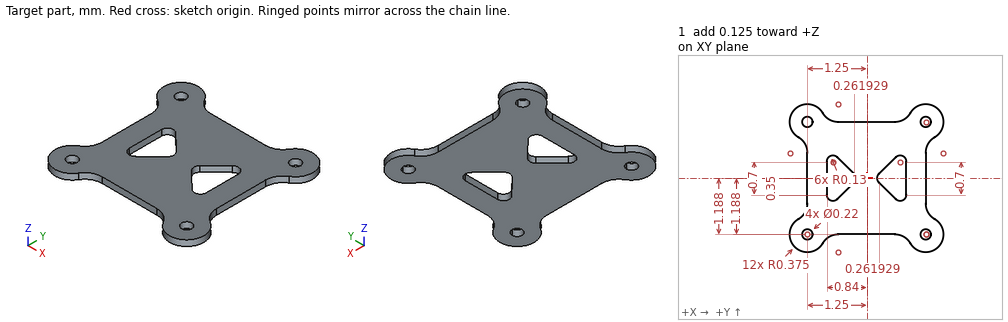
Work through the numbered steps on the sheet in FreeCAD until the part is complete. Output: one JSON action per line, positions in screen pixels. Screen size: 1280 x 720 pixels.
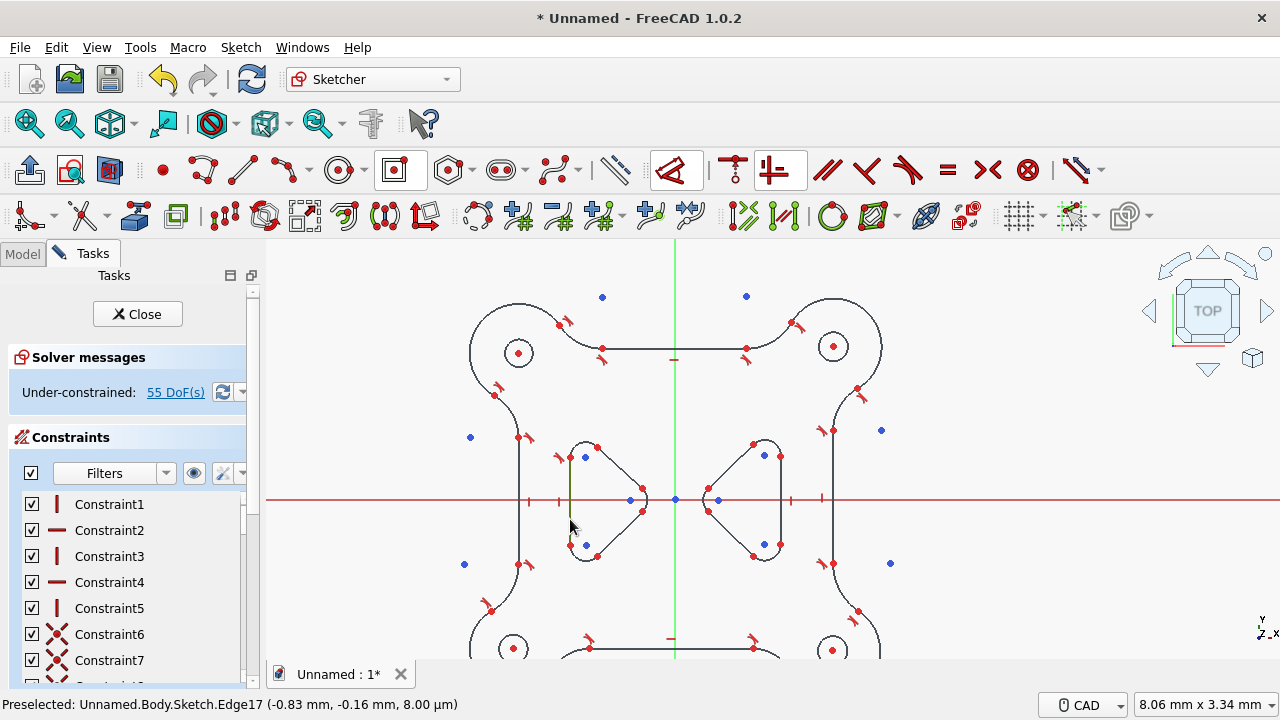
{"action": "scroll", "coordinate": [574, 556], "scroll_direction": "up", "scroll_amount": 2}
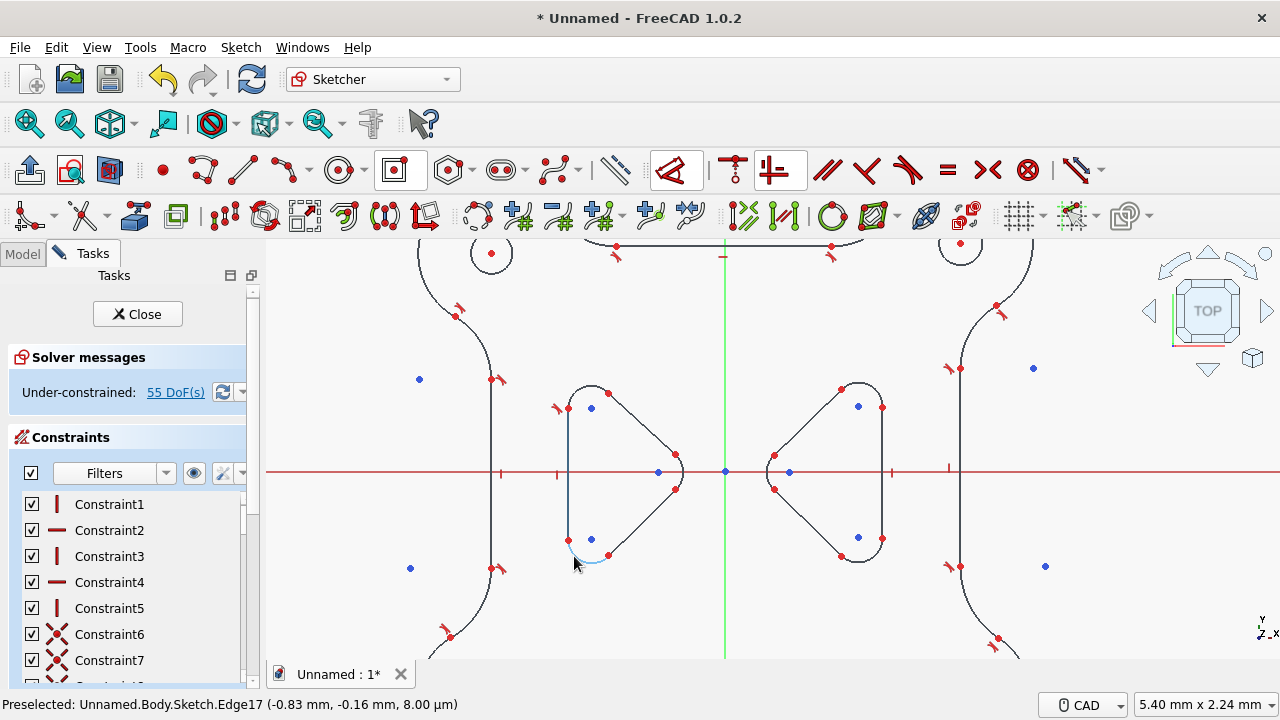
{"action": "left_click", "coordinate": [574, 555]}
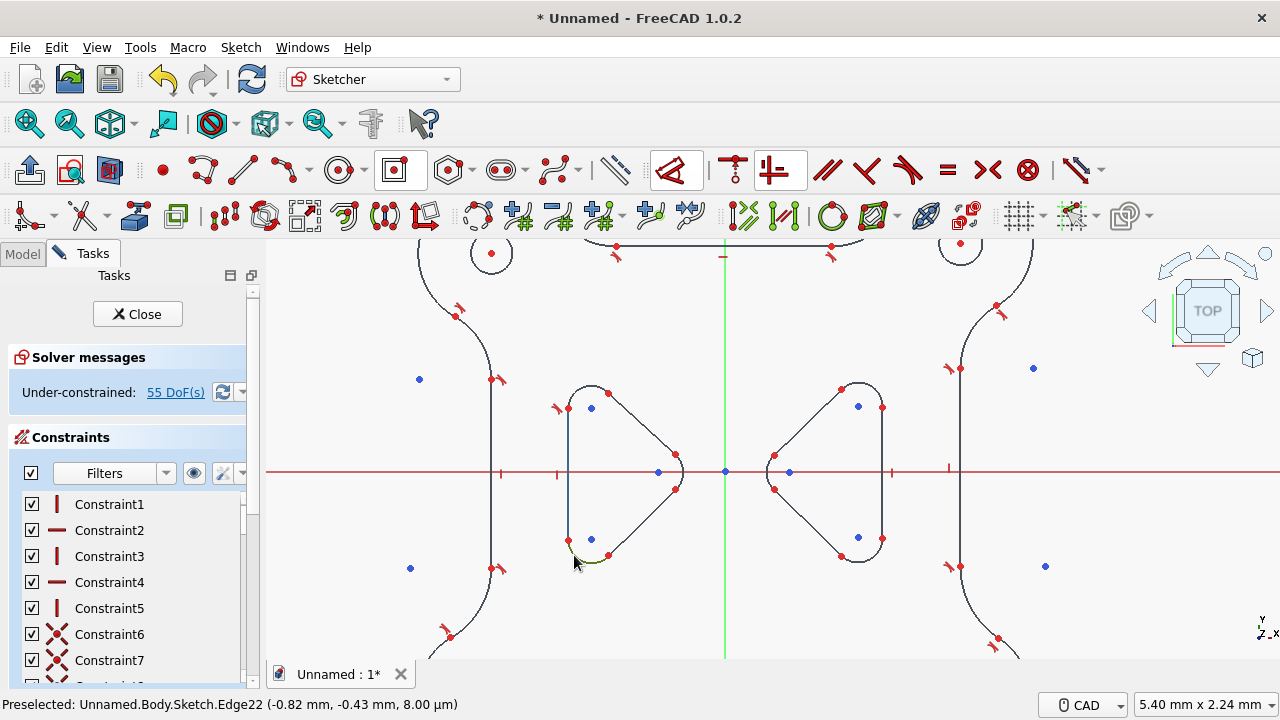
{"action": "left_click", "coordinate": [908, 170]}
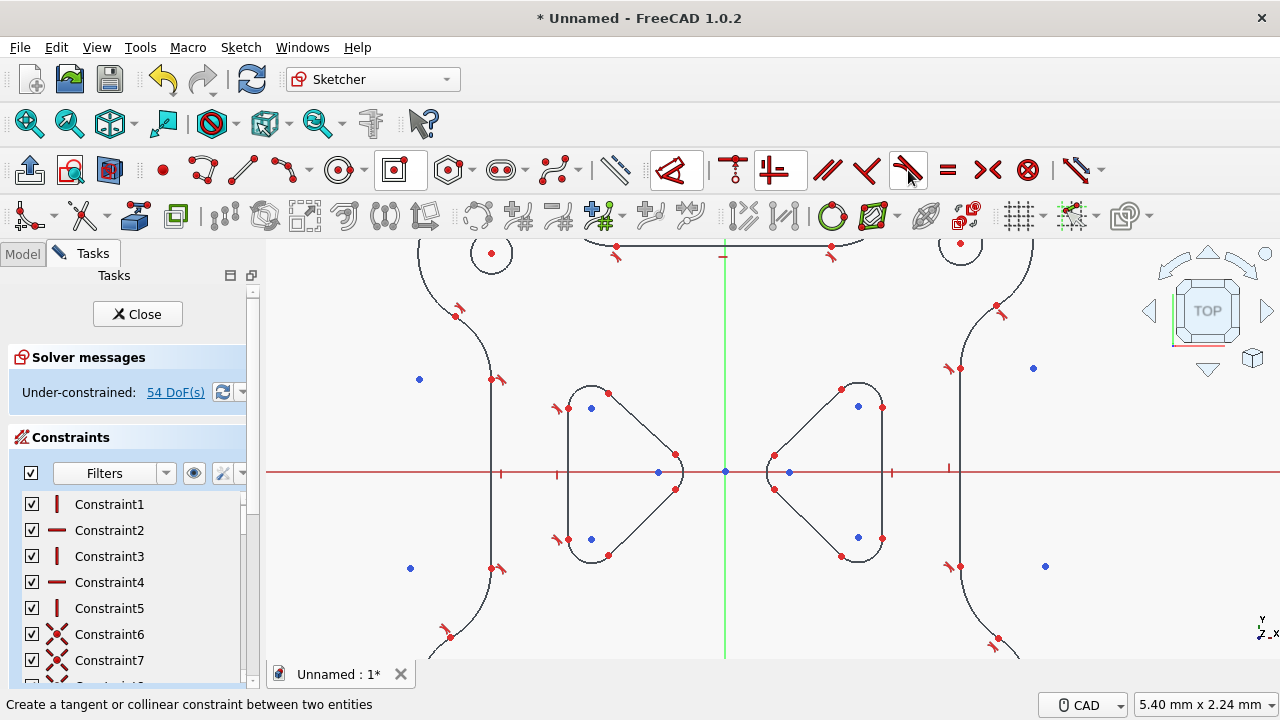
{"action": "left_click", "coordinate": [629, 412]}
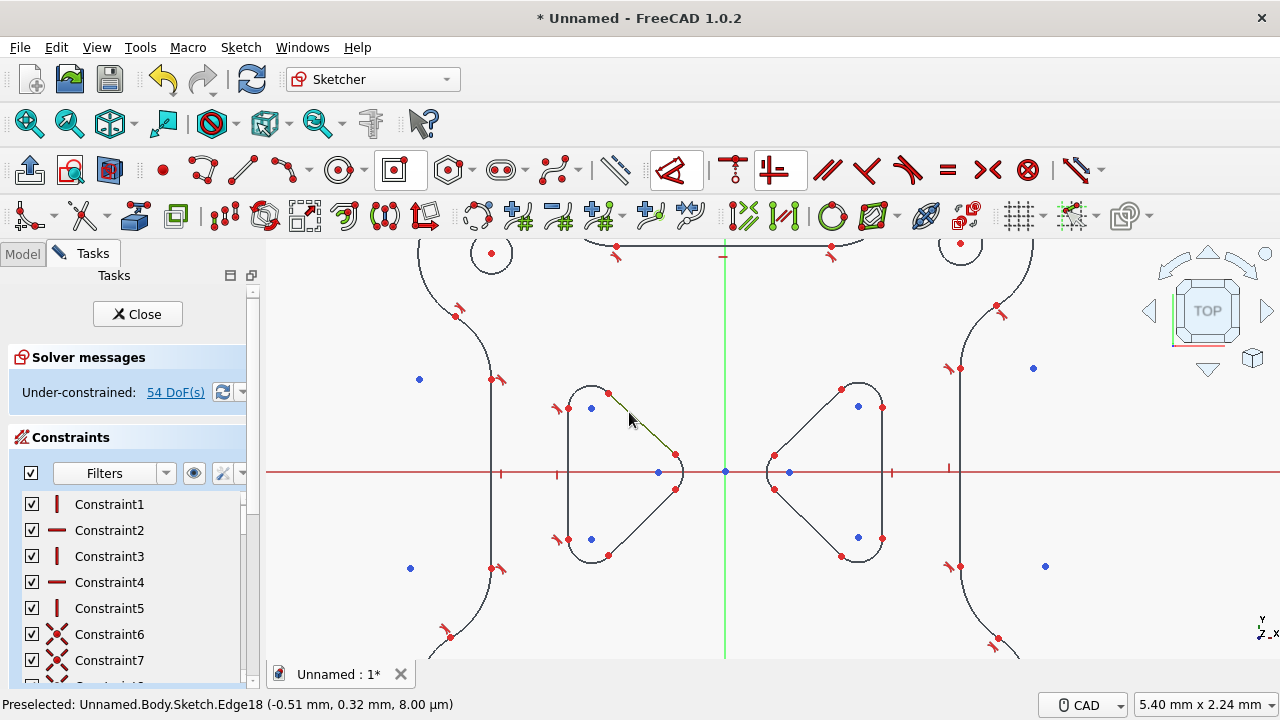
{"action": "left_click", "coordinate": [594, 386]}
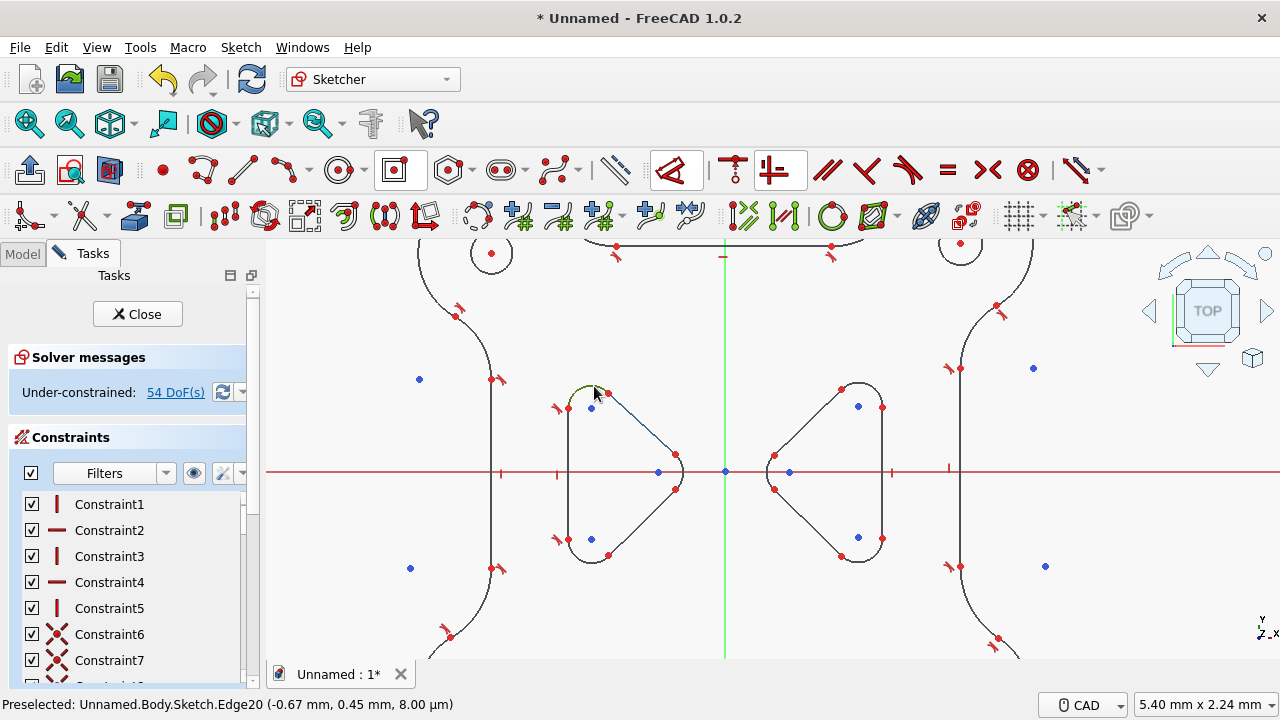
{"action": "left_click", "coordinate": [908, 170]}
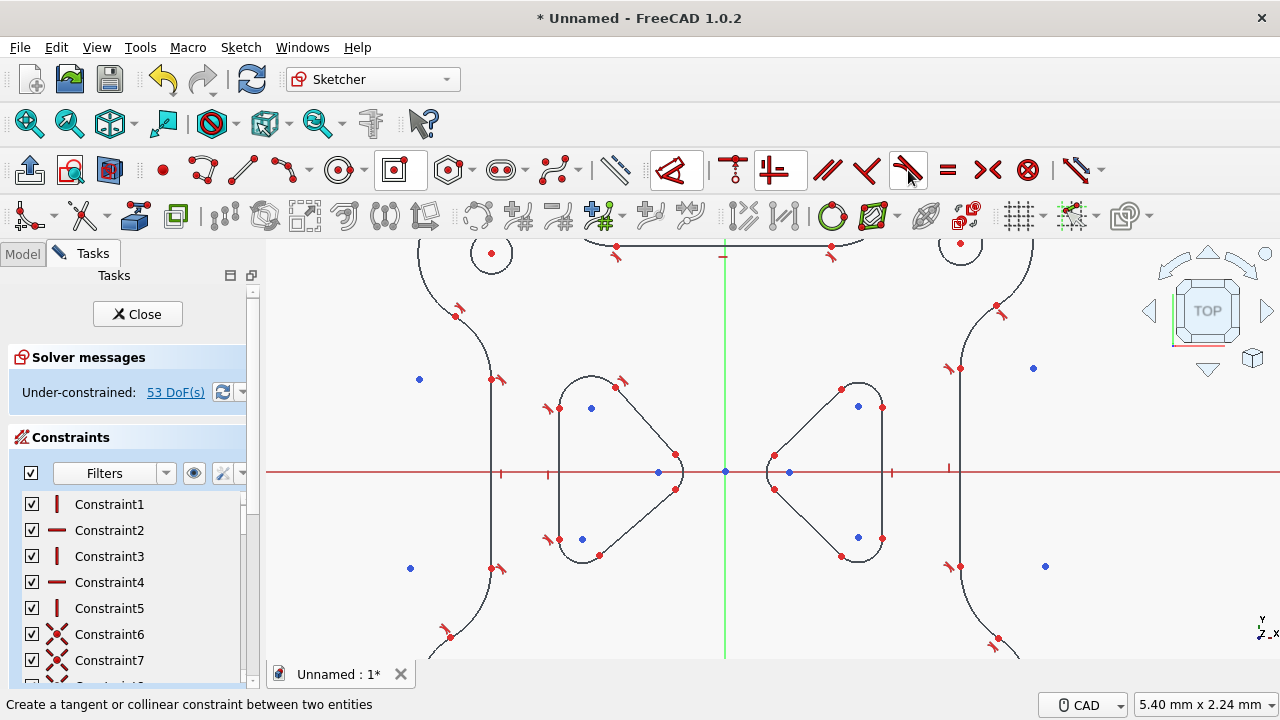
{"action": "left_click", "coordinate": [634, 408]}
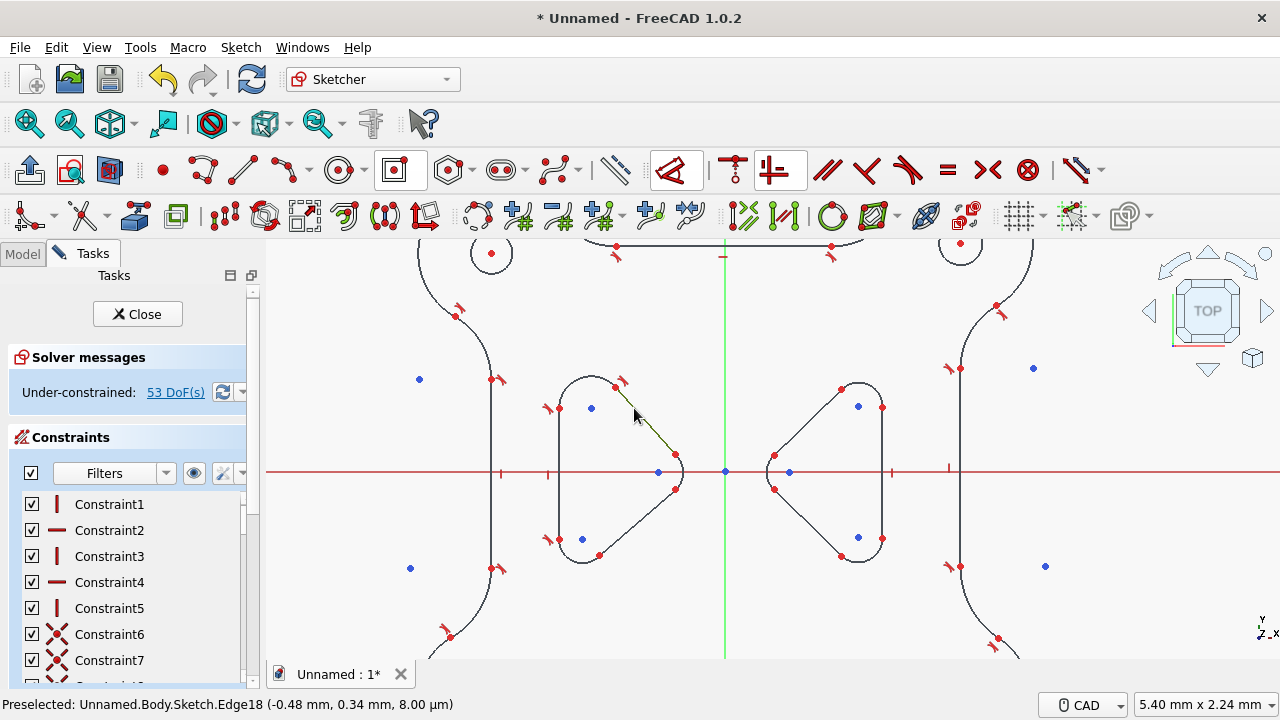
{"action": "left_click", "coordinate": [683, 472]}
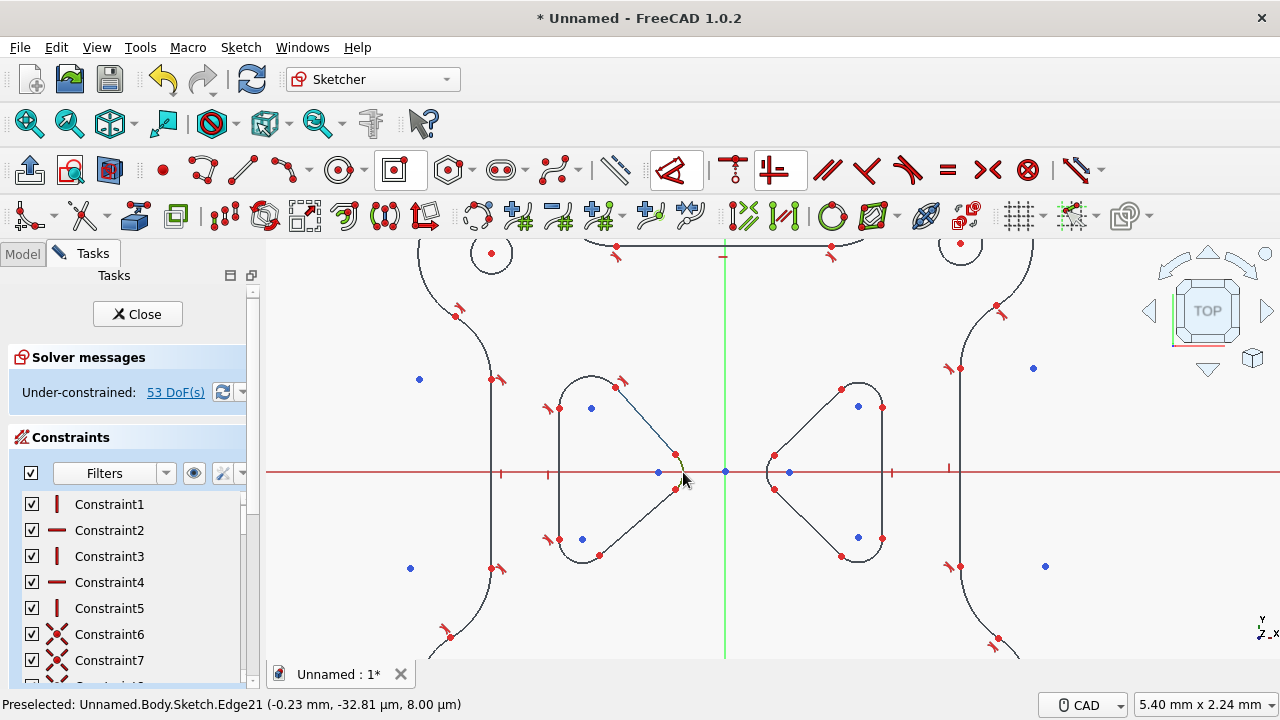
{"action": "left_click", "coordinate": [908, 170]}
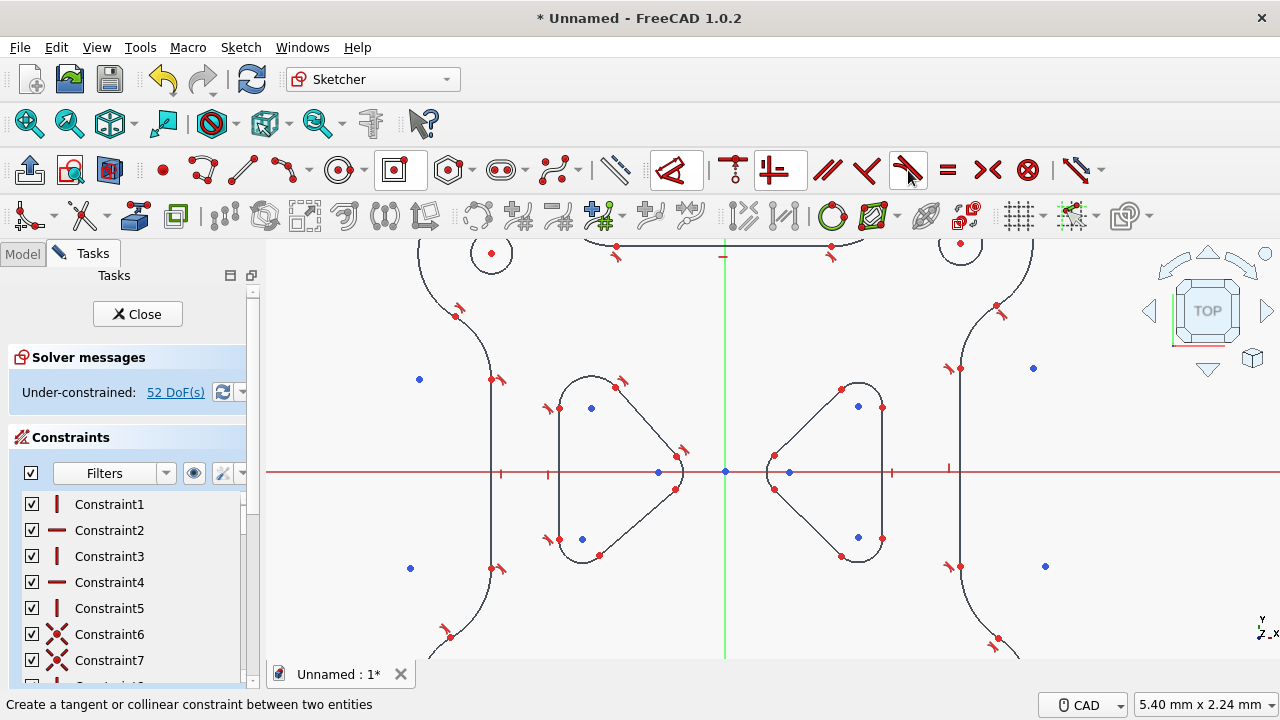
{"action": "left_click", "coordinate": [653, 510]}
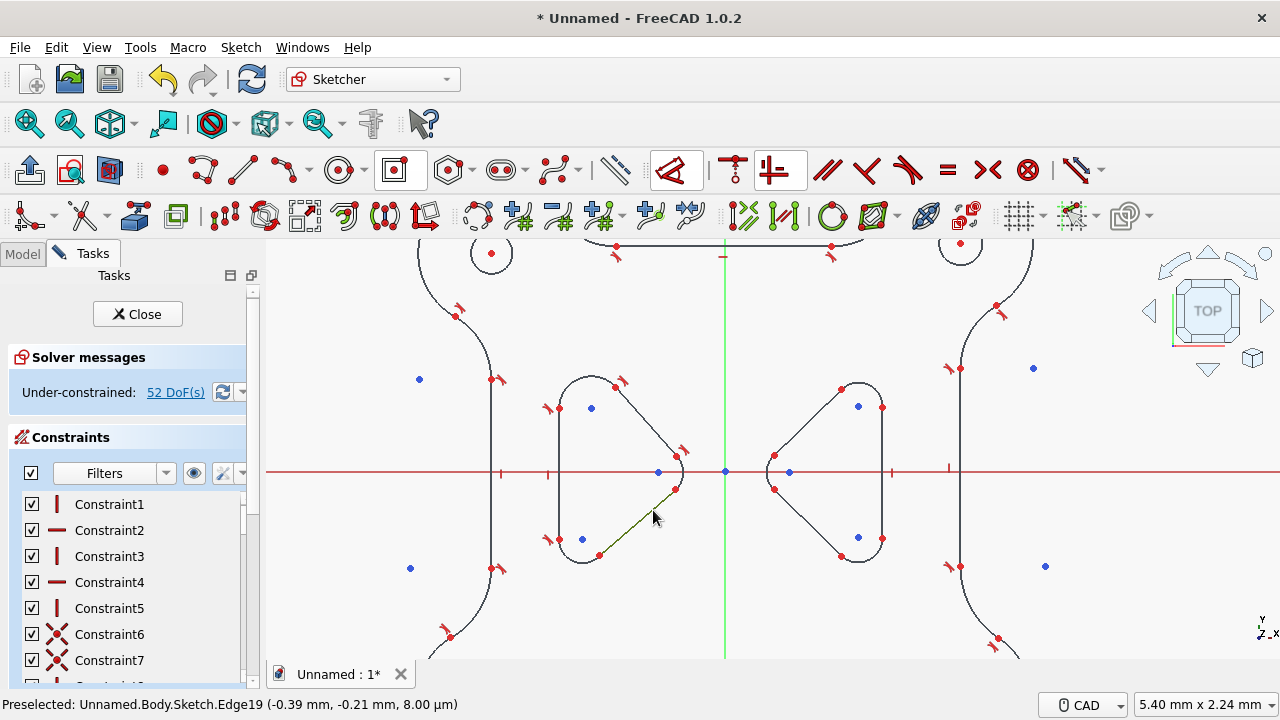
{"action": "left_click", "coordinate": [683, 473]}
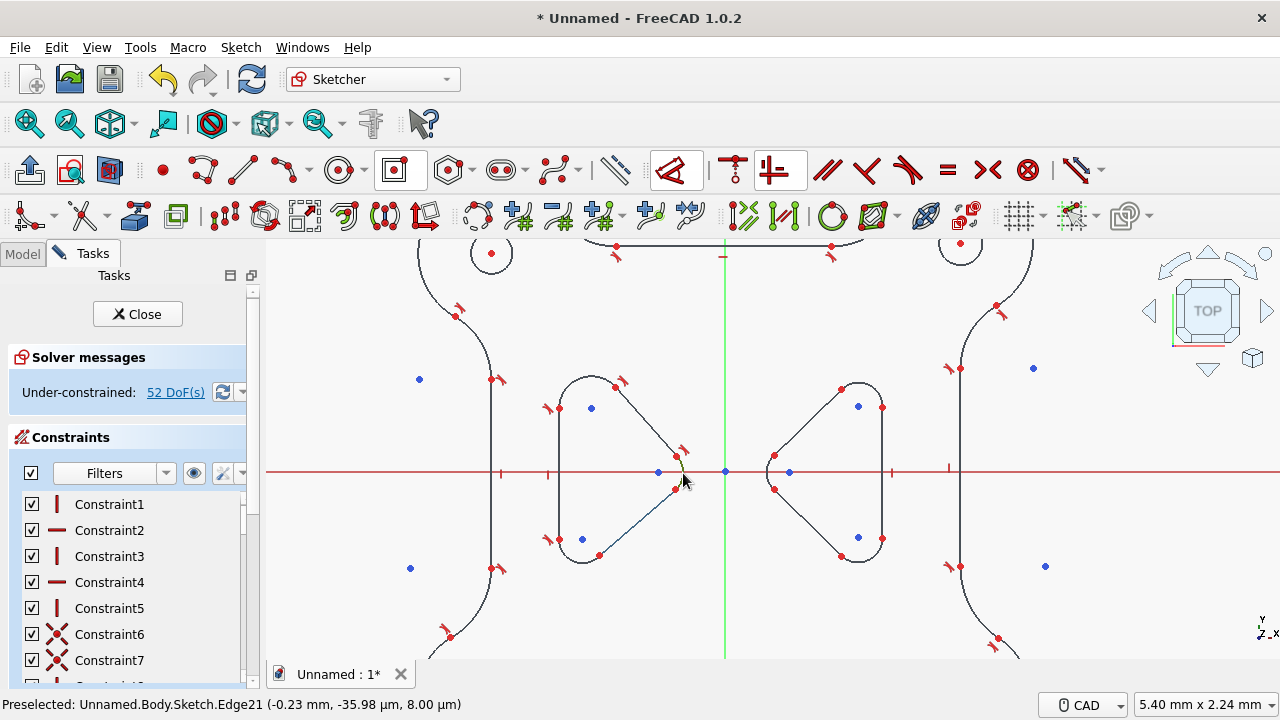
{"action": "left_click", "coordinate": [908, 170]}